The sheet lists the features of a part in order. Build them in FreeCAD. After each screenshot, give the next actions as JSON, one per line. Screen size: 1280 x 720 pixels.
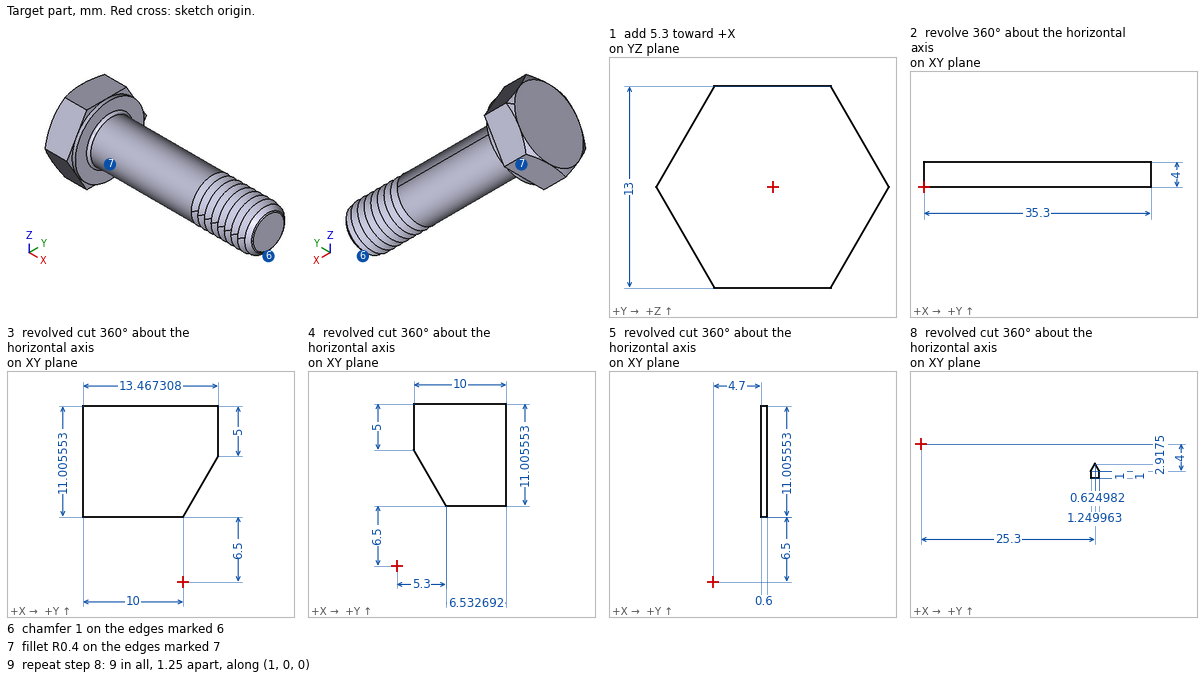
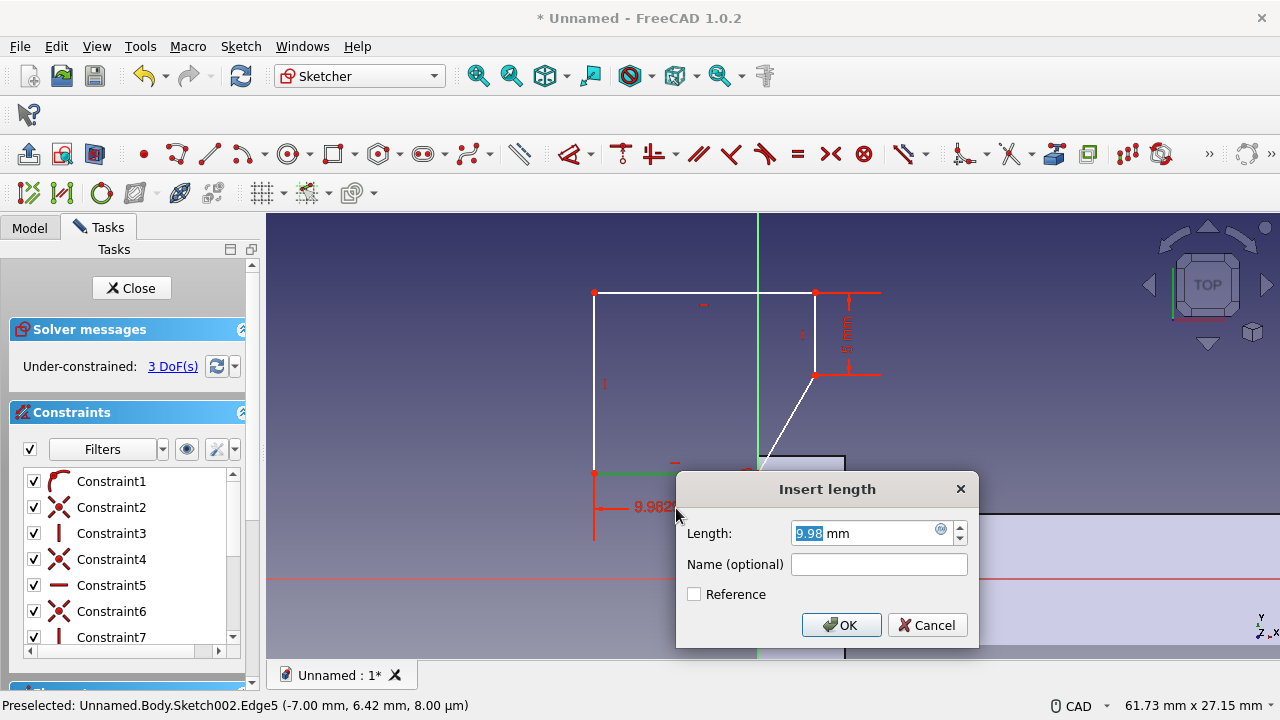
{"action": "type", "text": "10"}
{"action": "key", "text": "Return"}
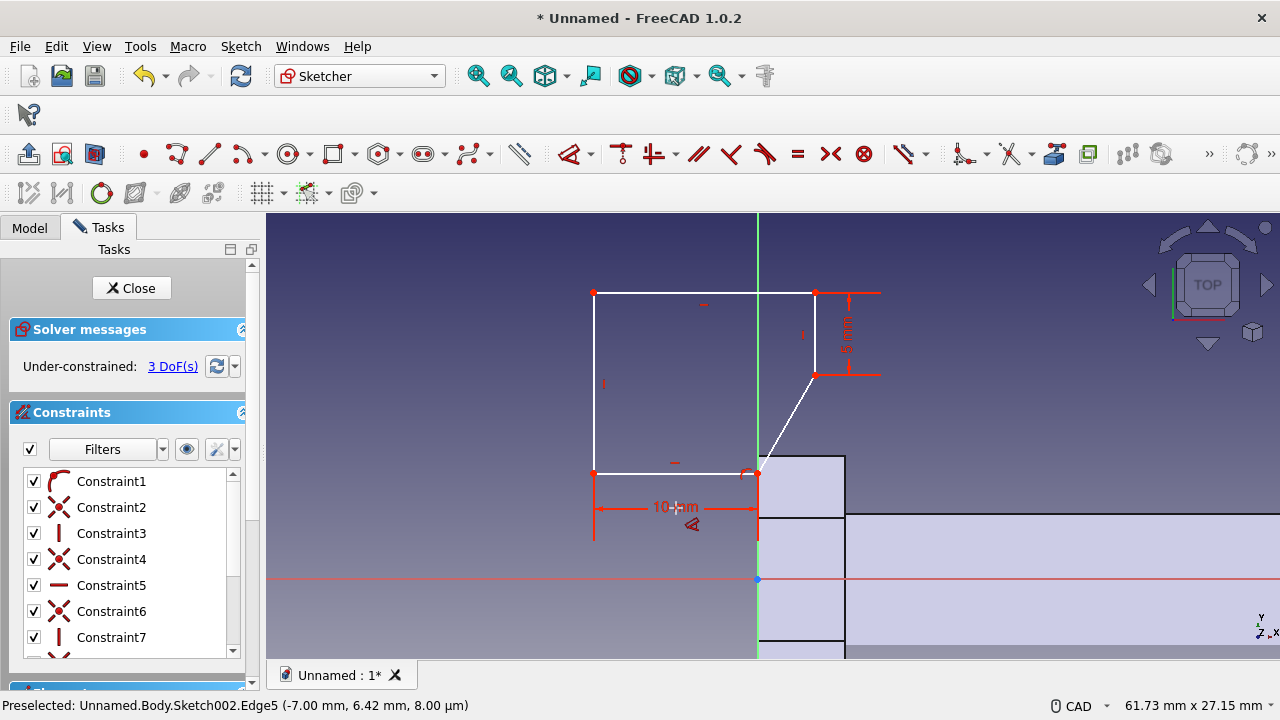
{"action": "left_click", "coordinate": [758, 474]}
{"action": "left_click", "coordinate": [792, 527]}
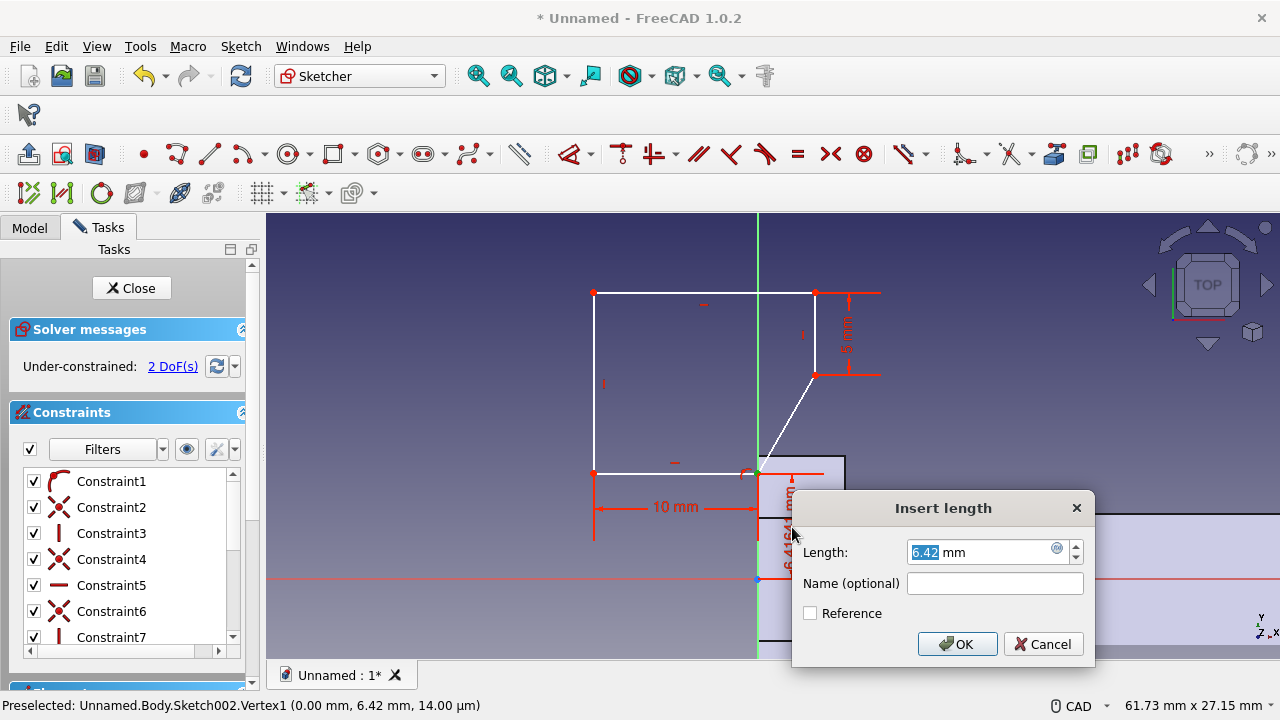
{"action": "type", "text": "6.5"}
{"action": "key", "text": "Return"}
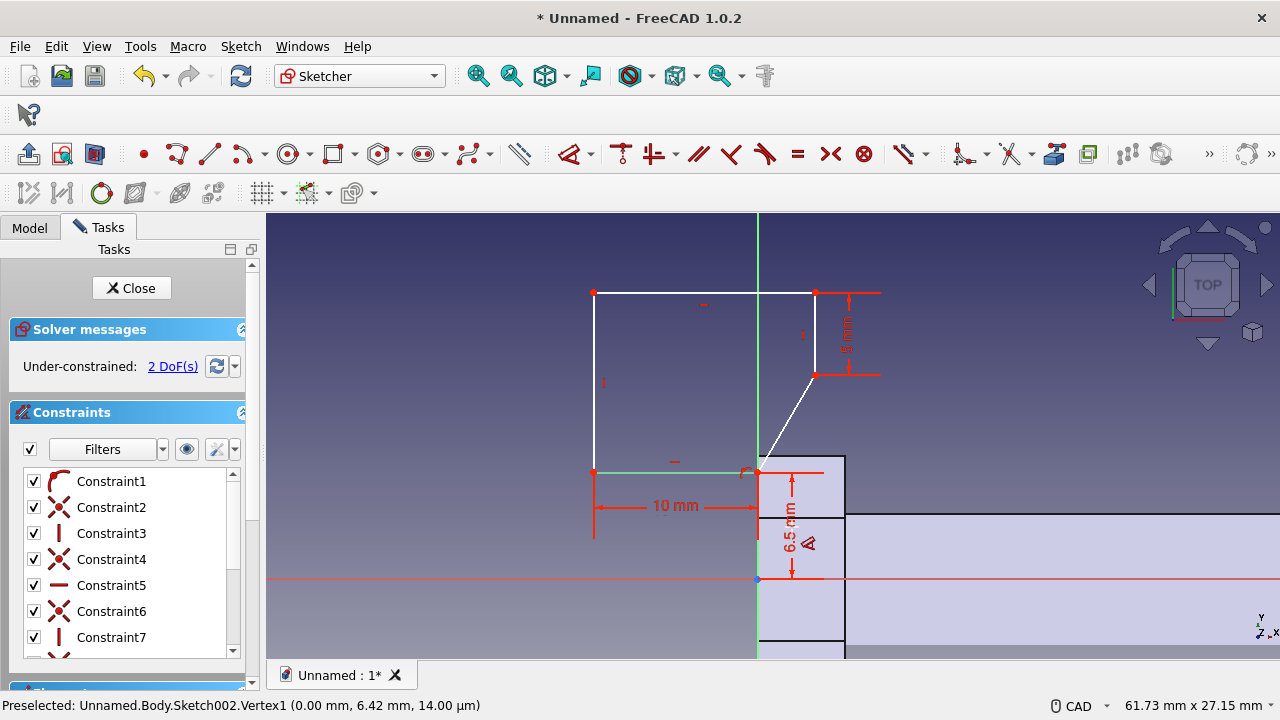
{"action": "scroll", "coordinate": [749, 293], "scroll_direction": "up", "scroll_amount": 2}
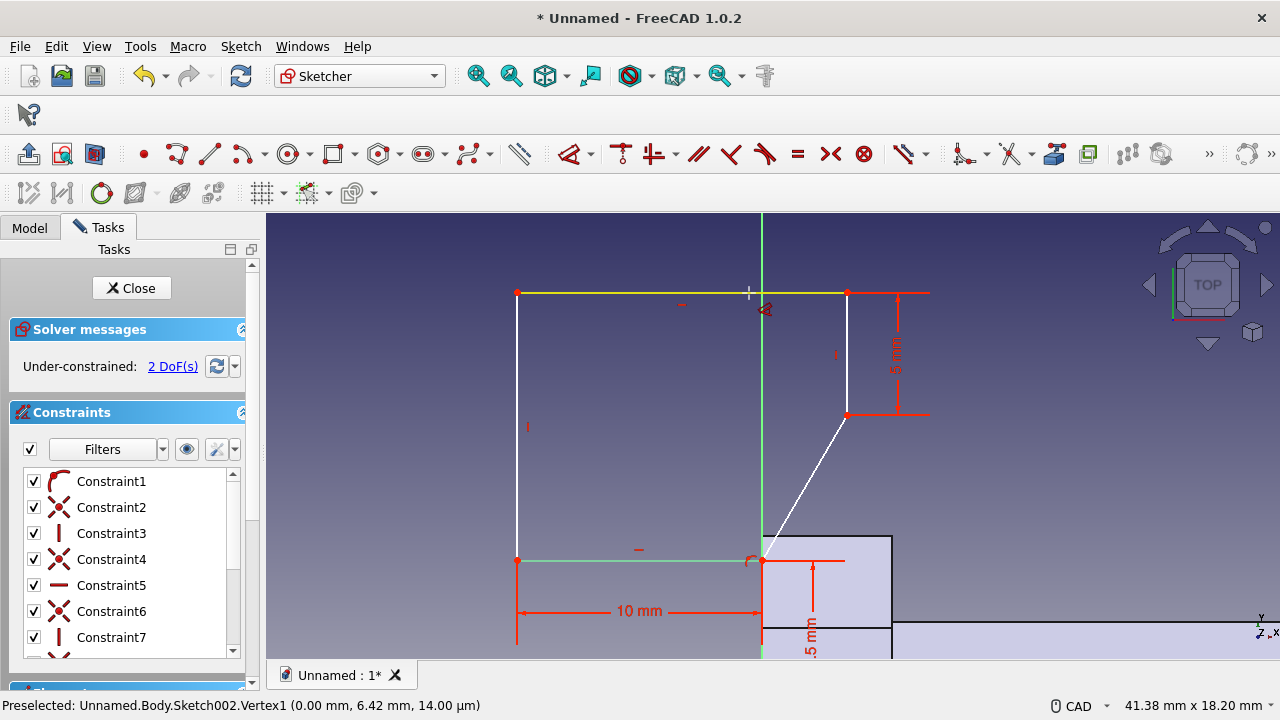
{"action": "left_click", "coordinate": [748, 293]}
{"action": "left_click", "coordinate": [682, 259]}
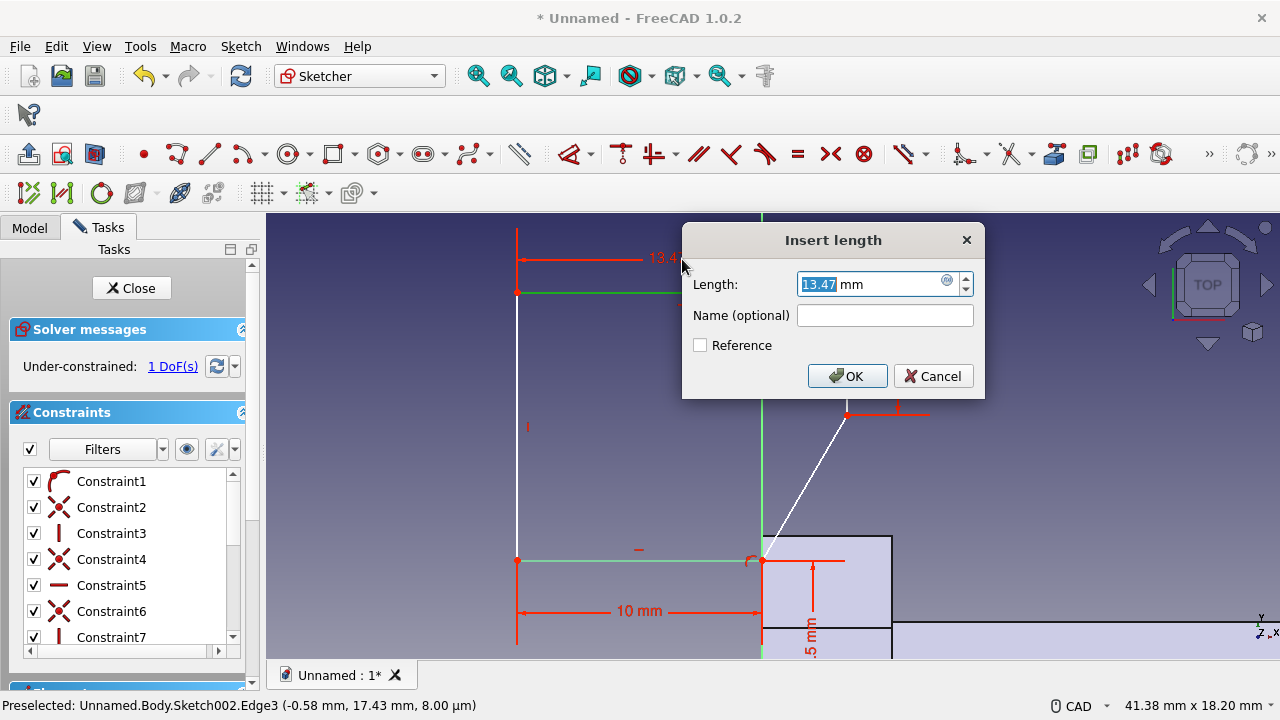
{"action": "type", "text": "13.467308"}
{"action": "key", "text": "Return"}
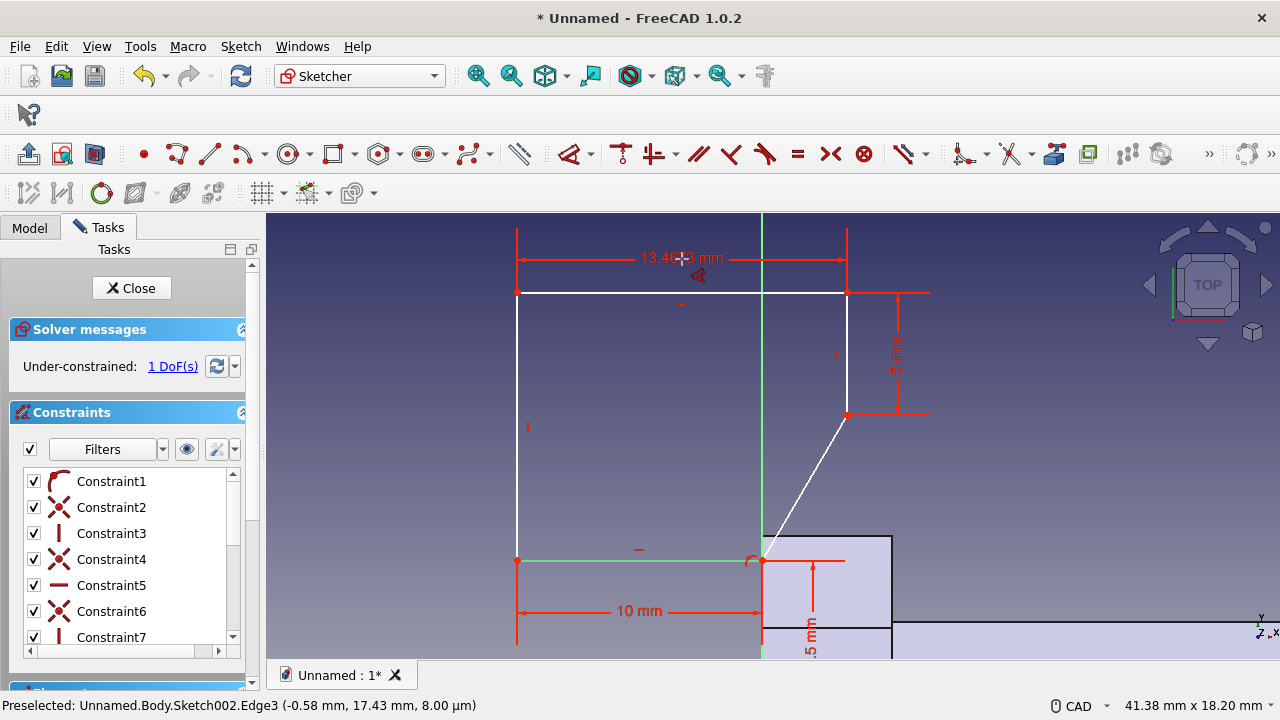
{"action": "left_click", "coordinate": [517, 373]}
{"action": "left_click", "coordinate": [483, 427]}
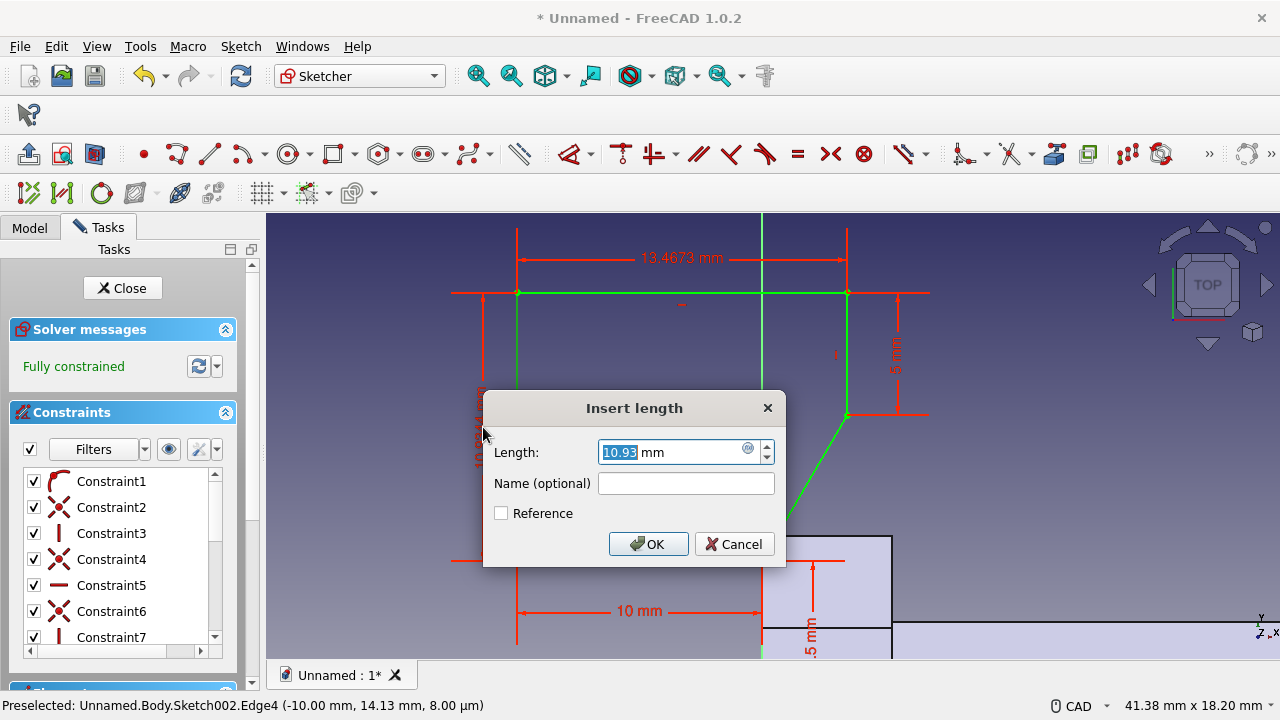
{"action": "type", "text": "11.005553"}
{"action": "key", "text": "Return"}
{"action": "key", "text": "Escape"}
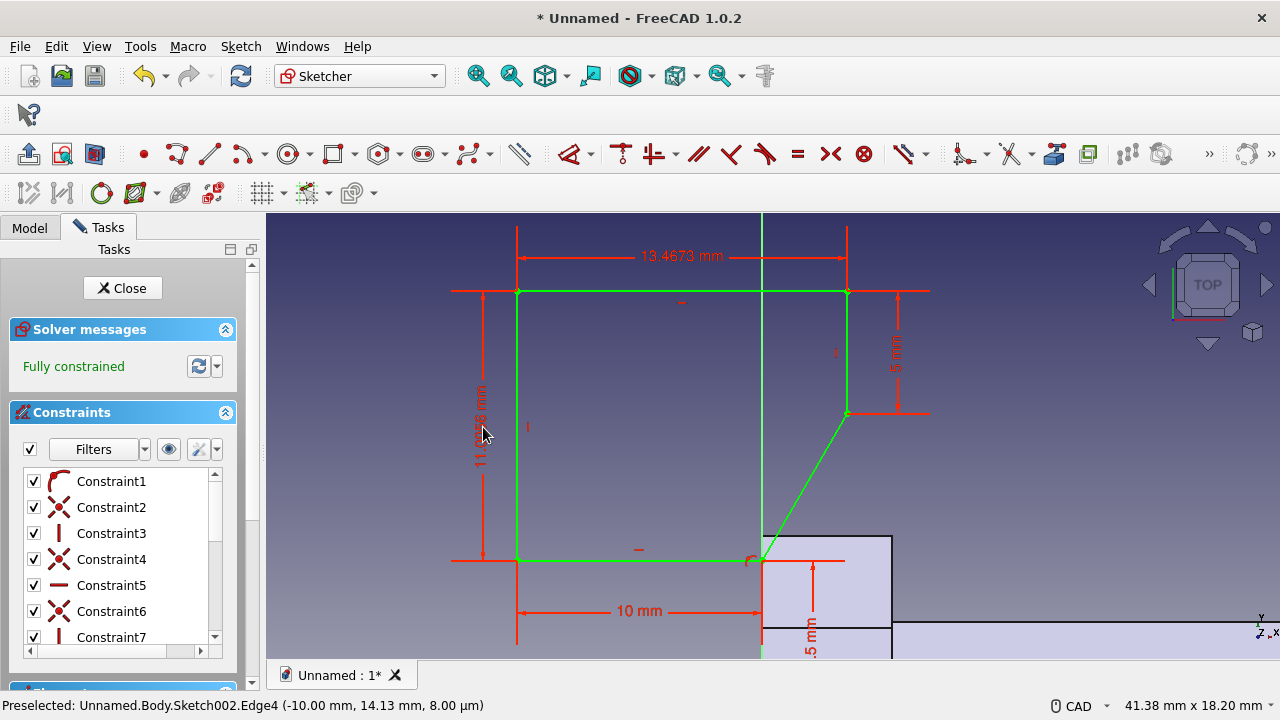
{"action": "left_click", "coordinate": [123, 288]}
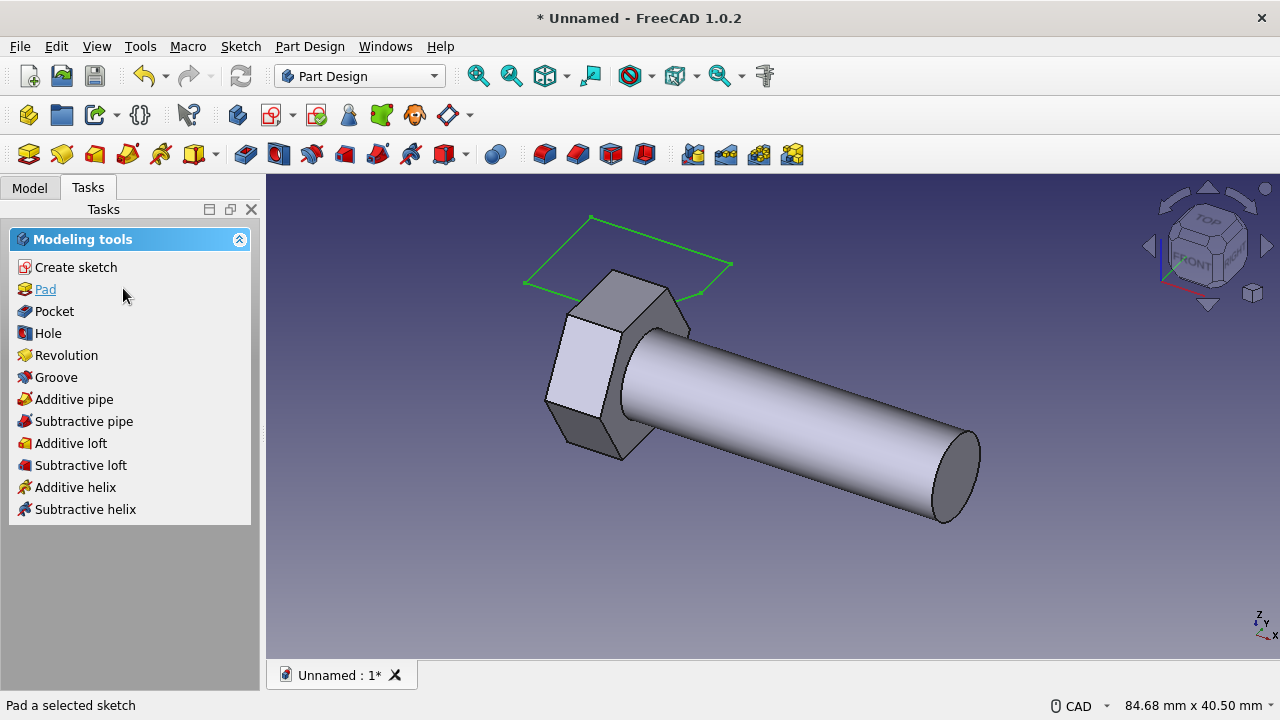
{"action": "left_click", "coordinate": [312, 154]}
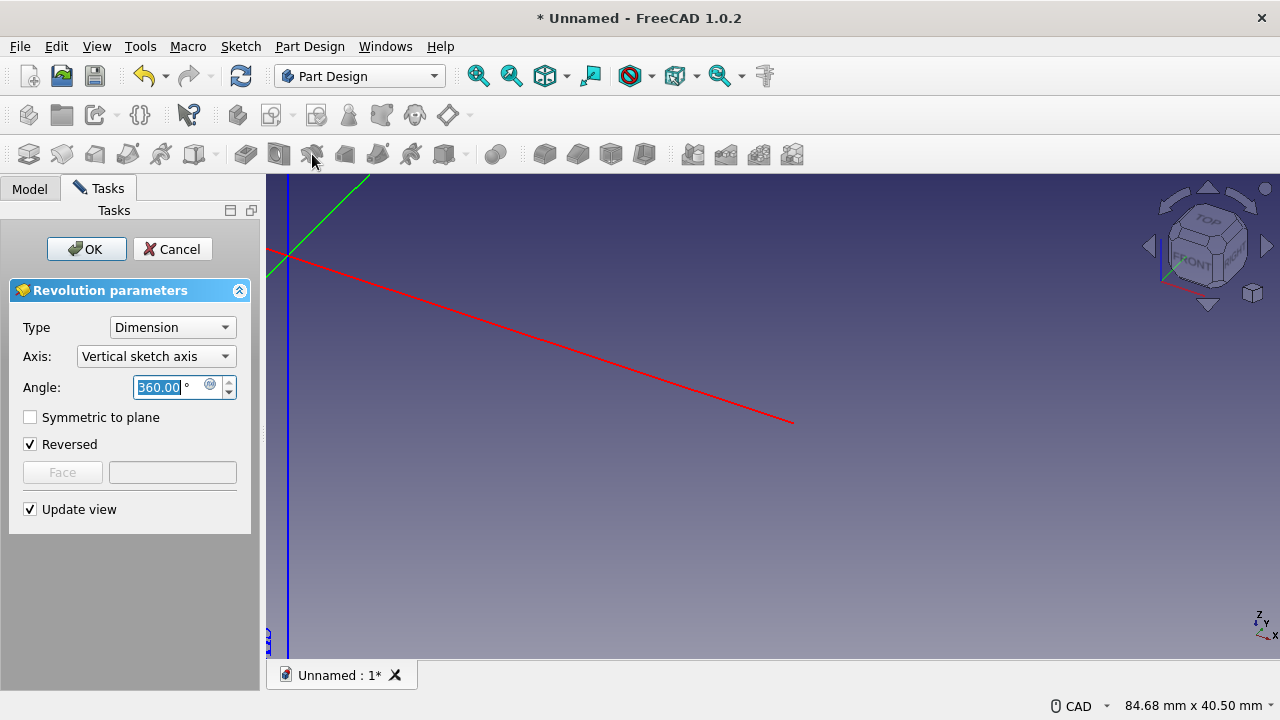
{"action": "left_click", "coordinate": [157, 356]}